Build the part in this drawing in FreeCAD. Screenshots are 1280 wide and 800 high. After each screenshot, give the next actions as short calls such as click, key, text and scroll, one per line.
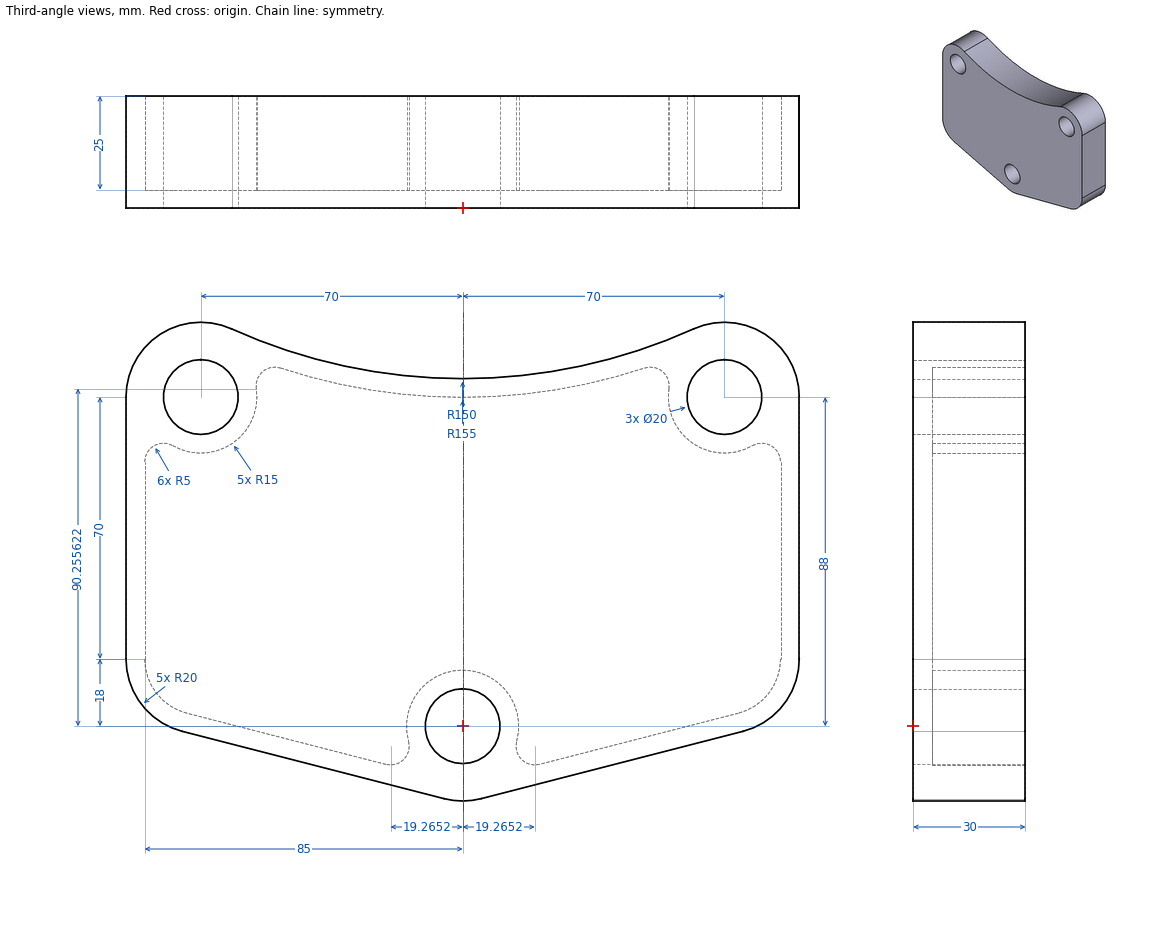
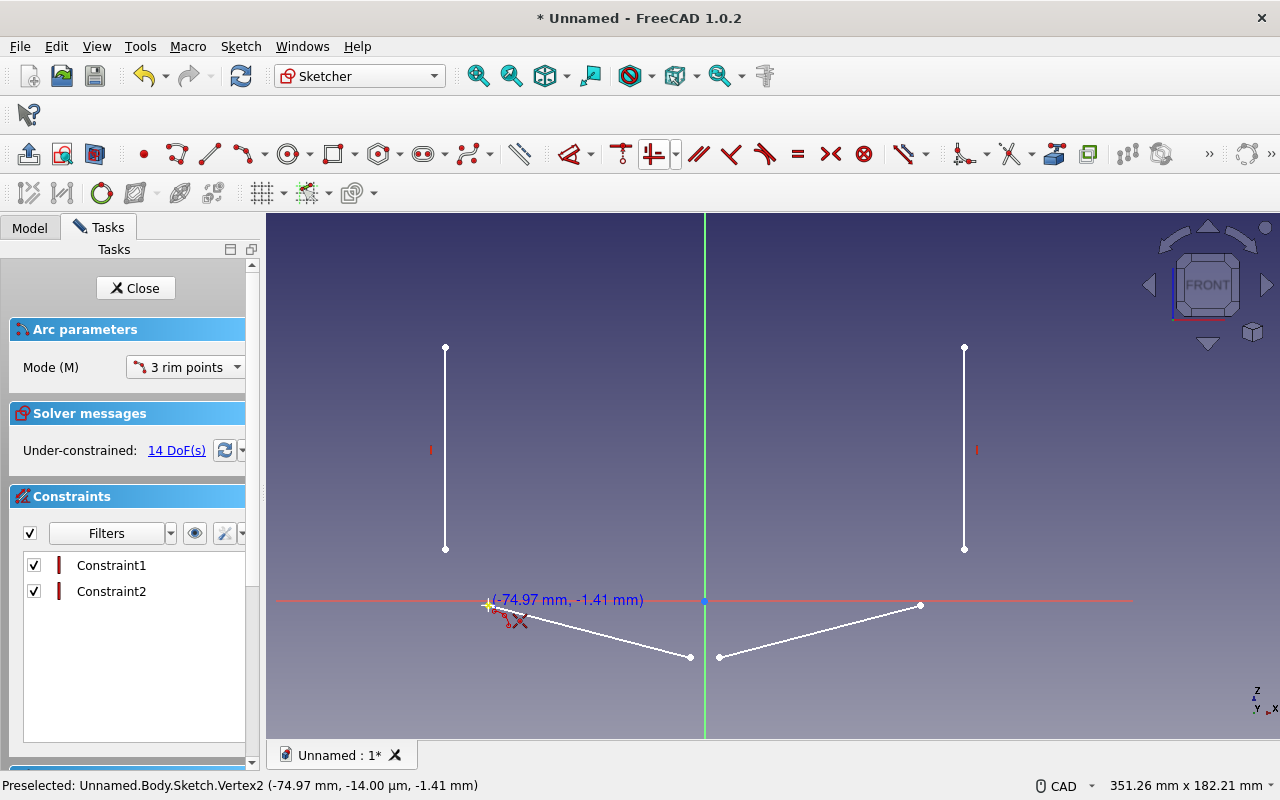
click(445, 550)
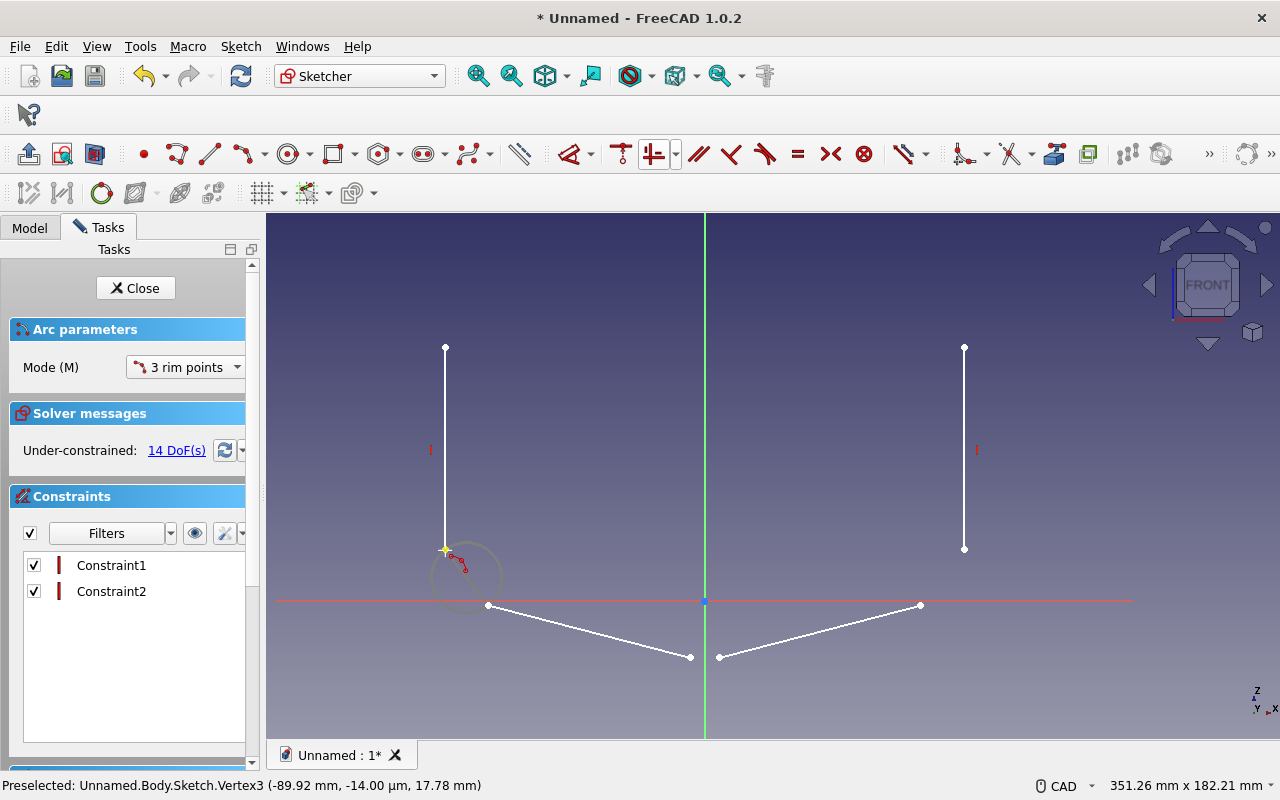
scroll(457, 585, up, 2)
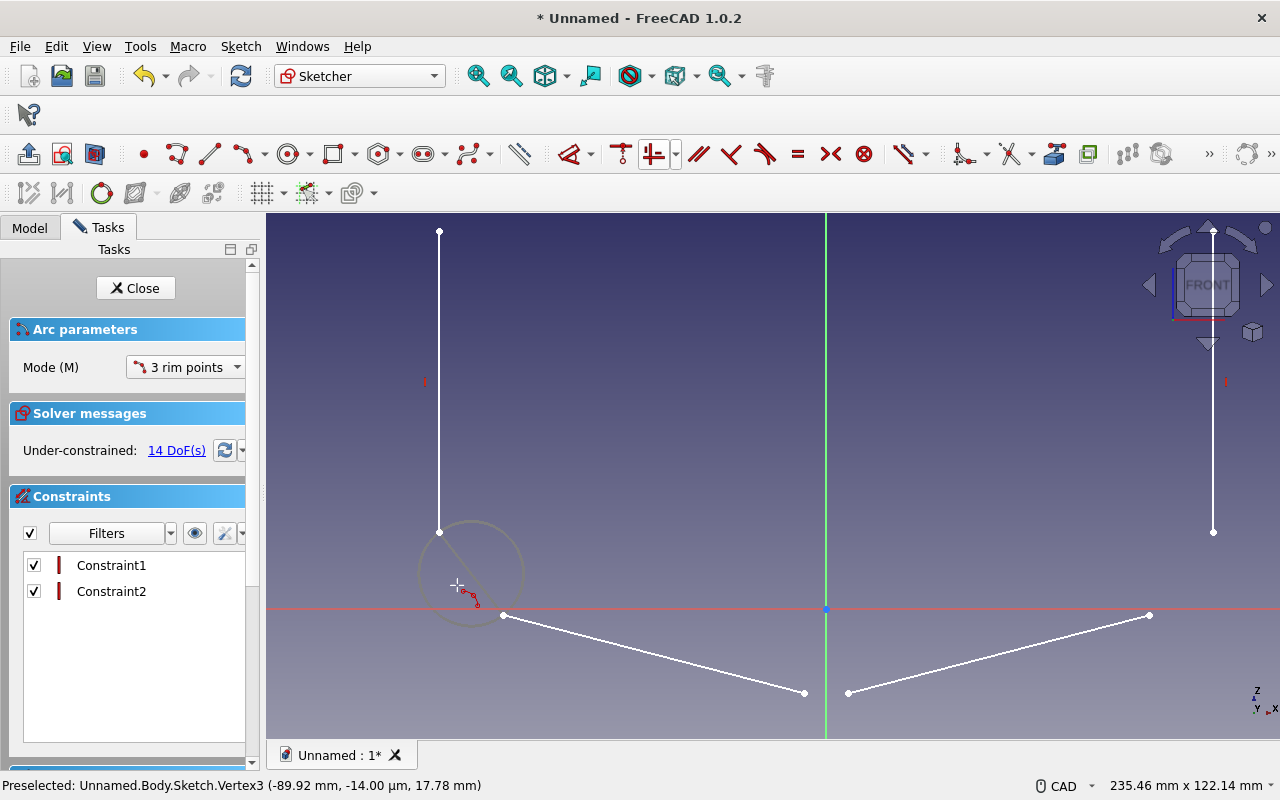
click(457, 584)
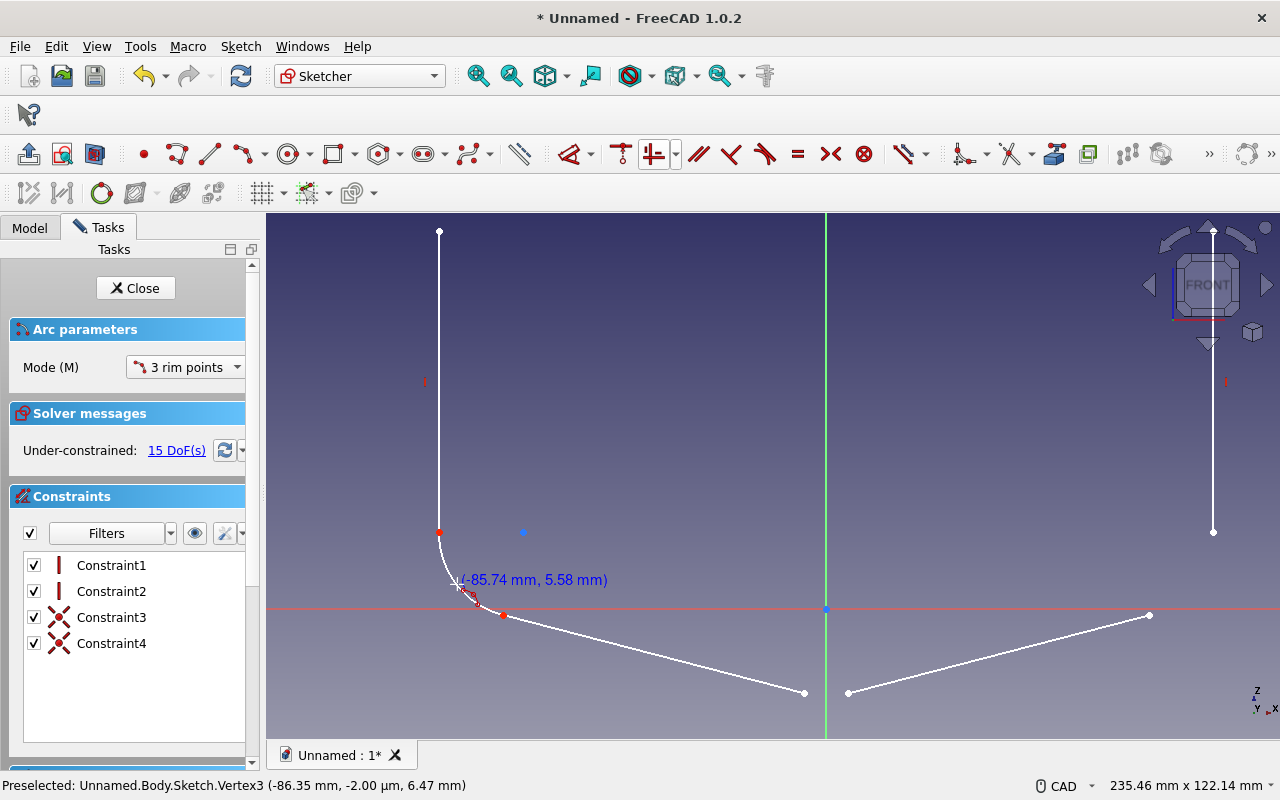
scroll(457, 583, down, 2)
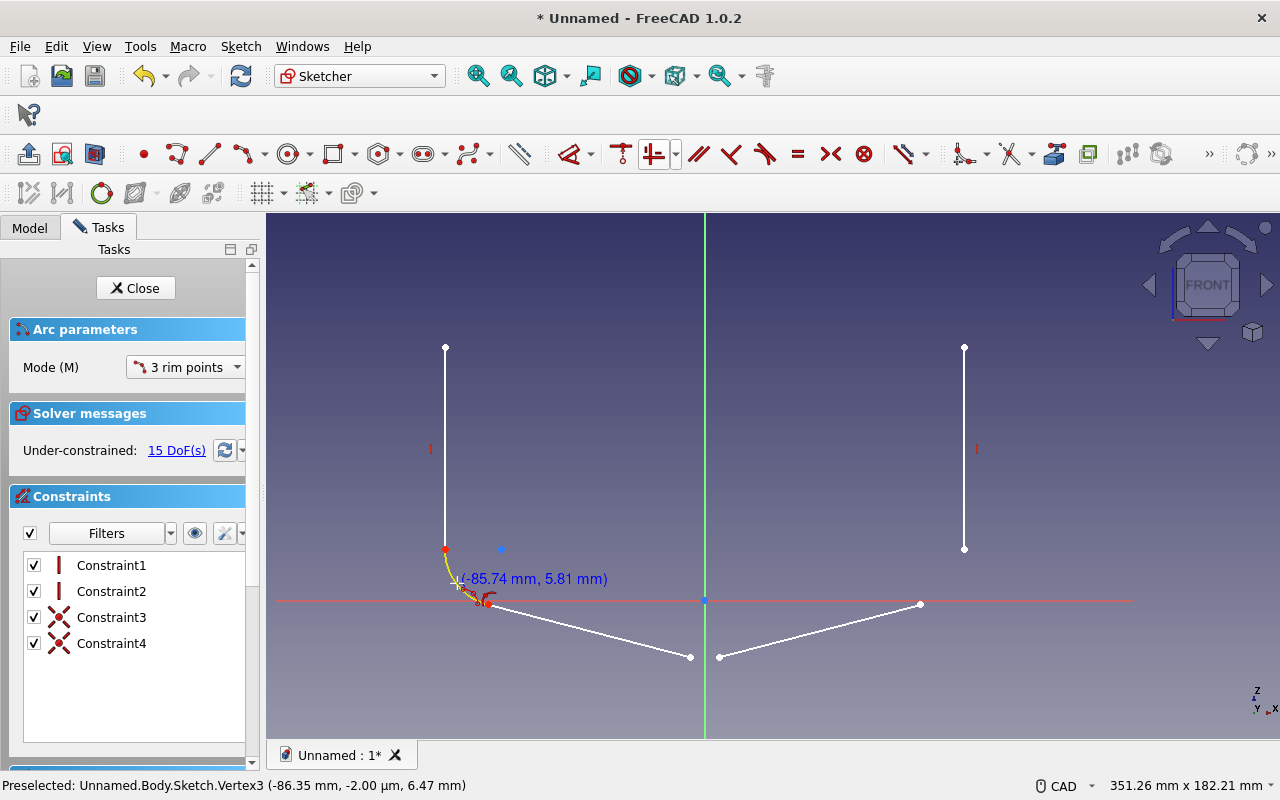
click(445, 347)
click(526, 294)
click(471, 298)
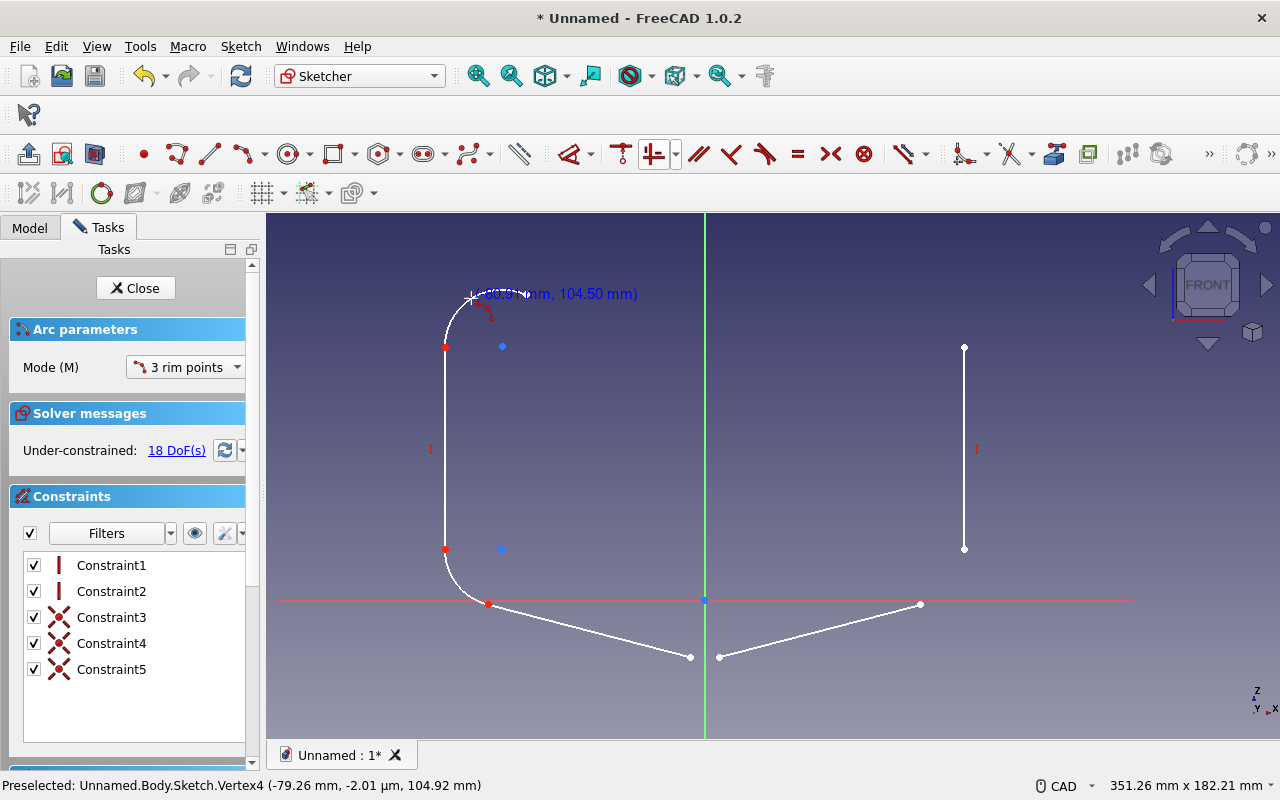
click(526, 295)
click(883, 294)
click(668, 331)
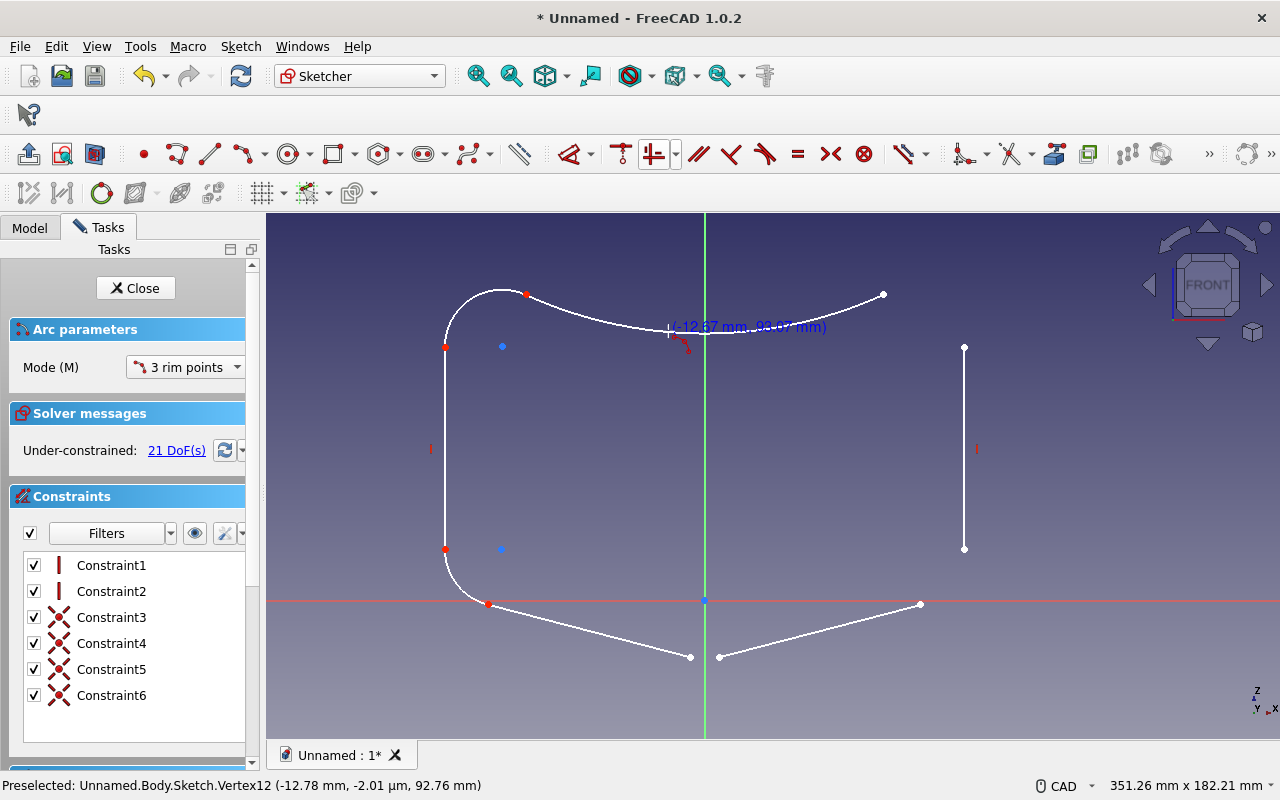
click(883, 295)
click(964, 347)
click(938, 298)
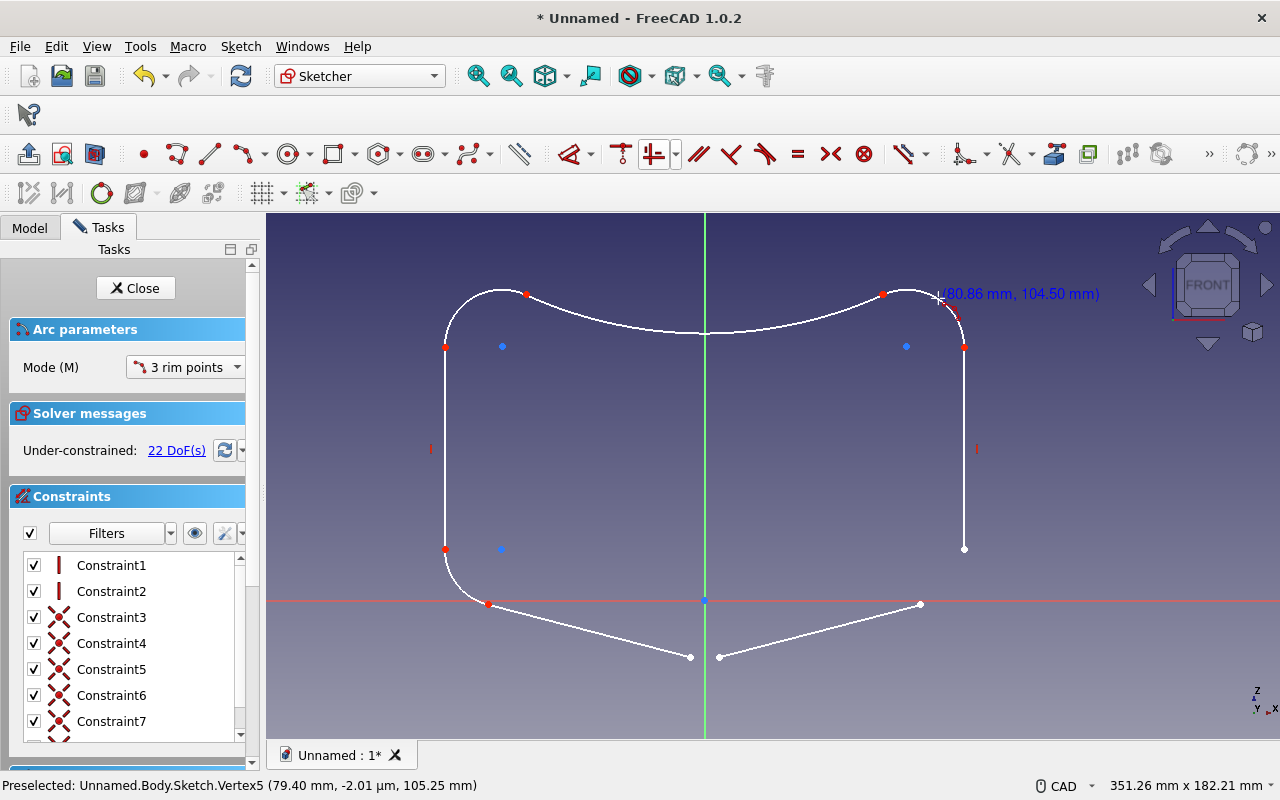
click(964, 549)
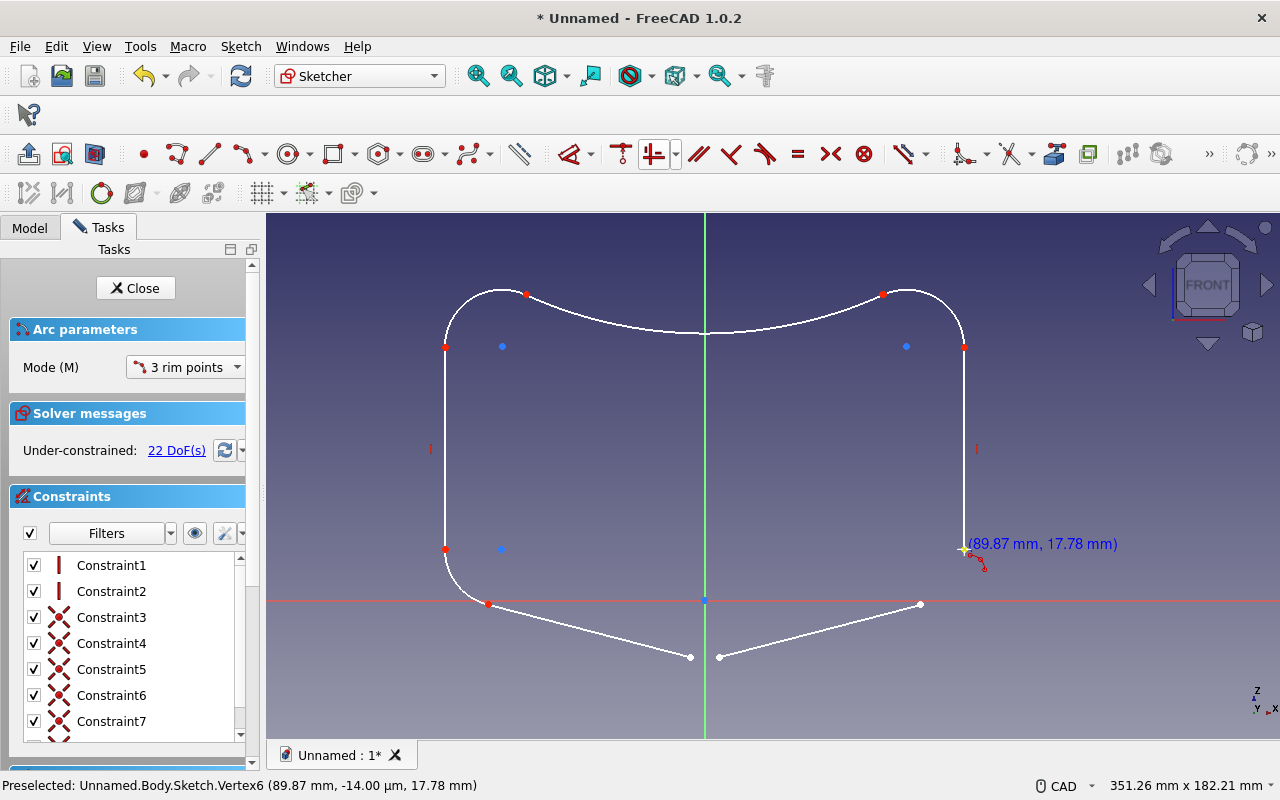
scroll(921, 605, up, 7)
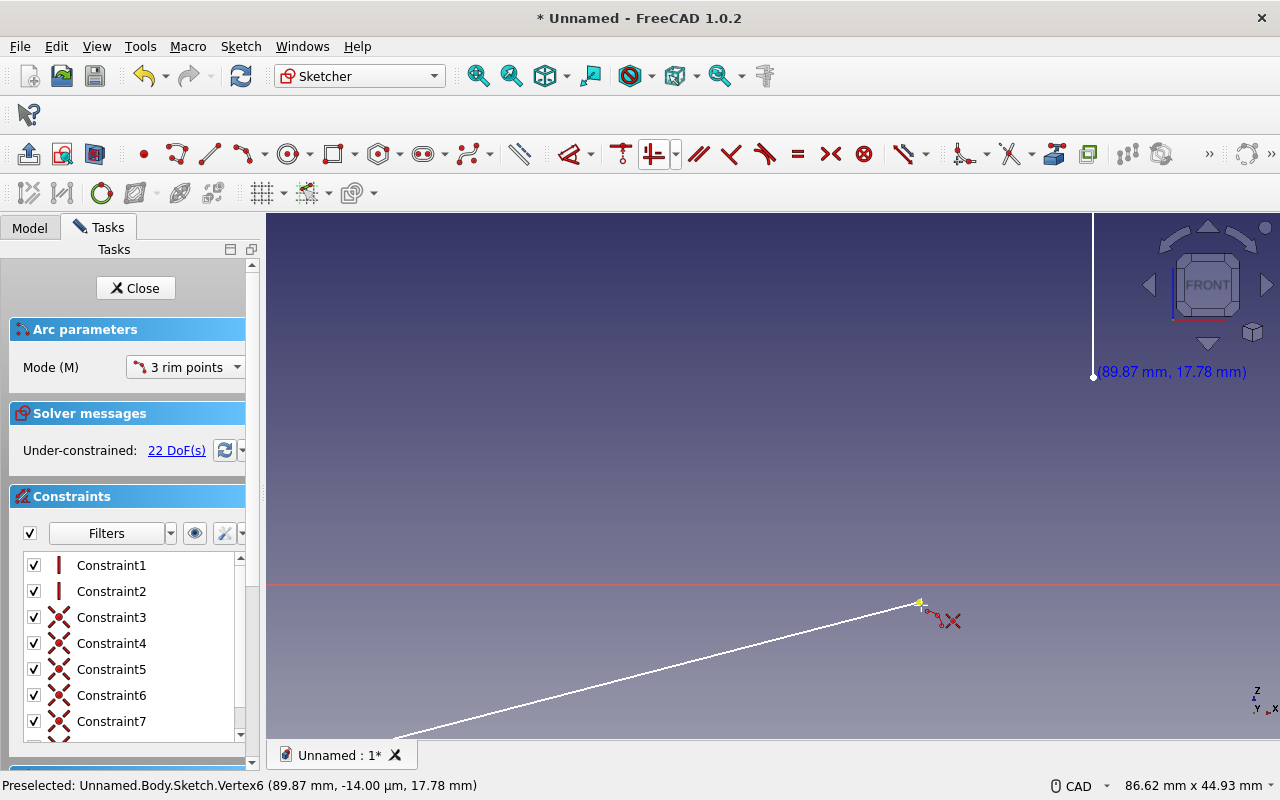
click(919, 602)